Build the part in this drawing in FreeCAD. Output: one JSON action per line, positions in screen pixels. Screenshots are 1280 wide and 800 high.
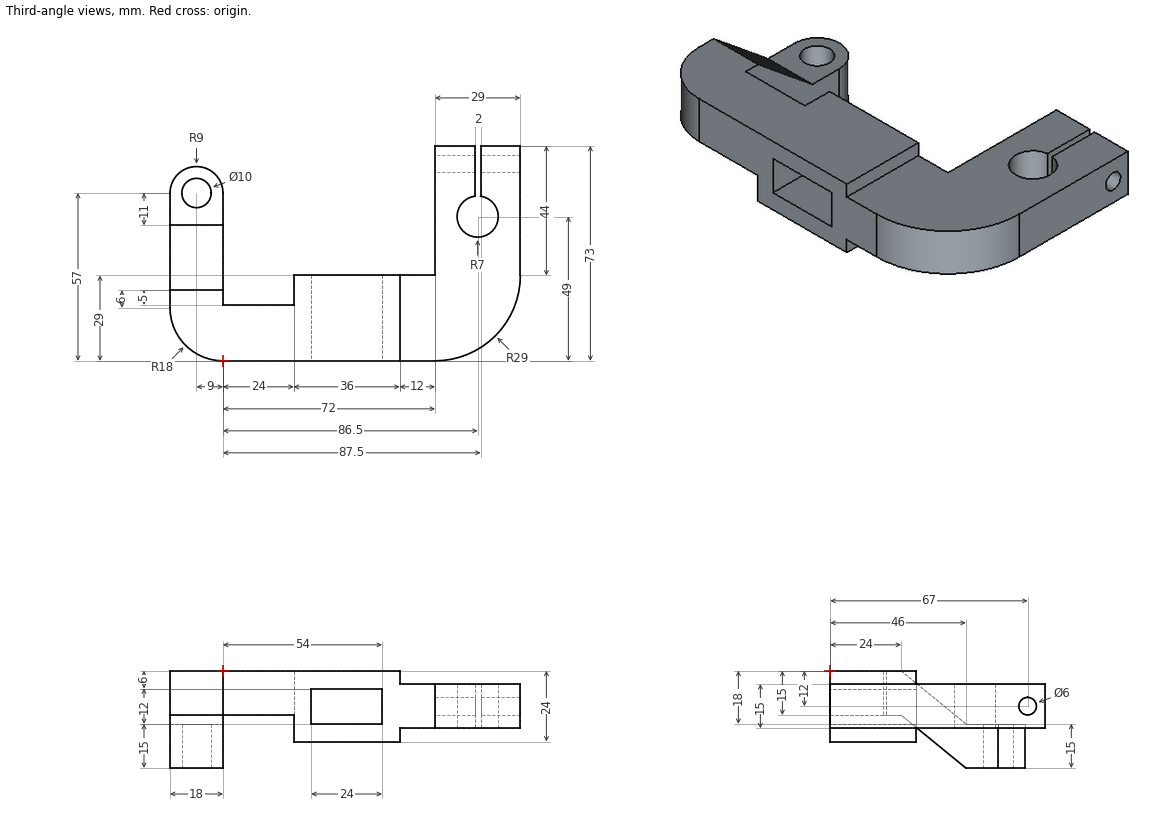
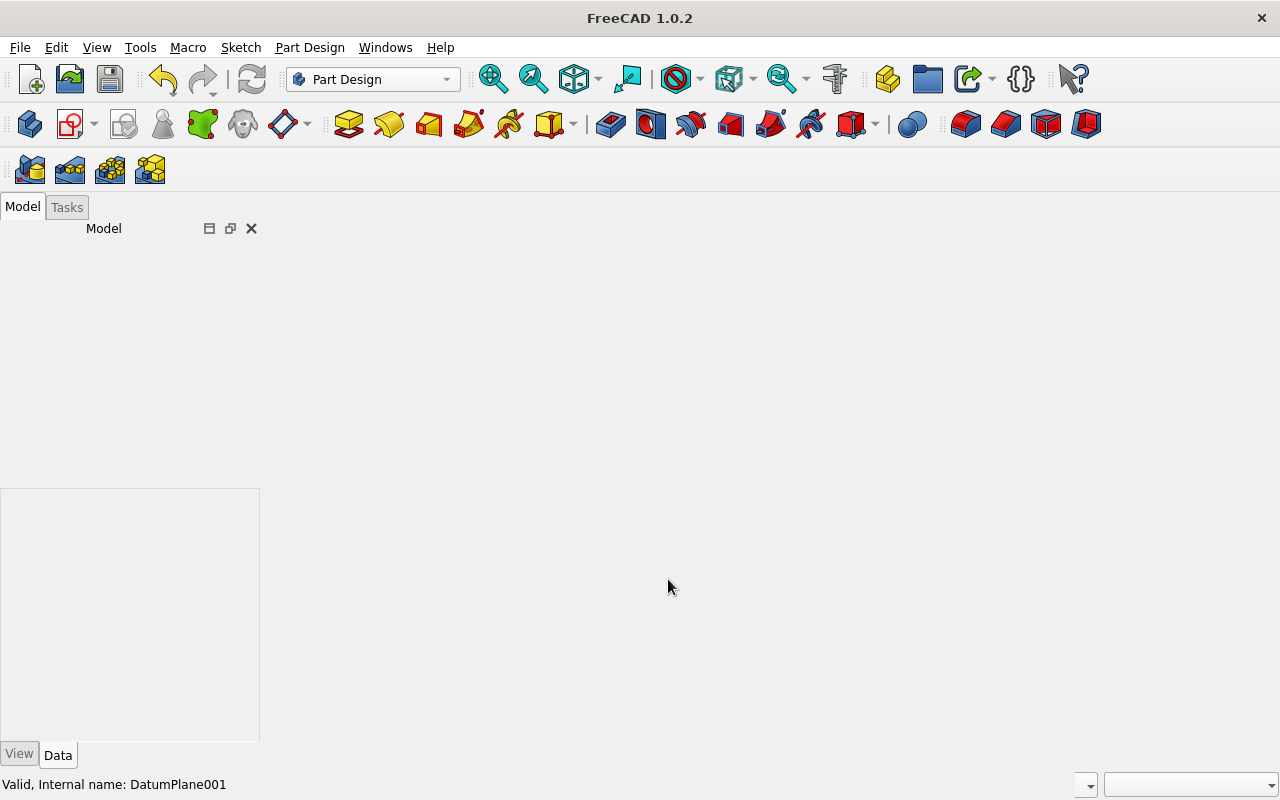
{"action": "key", "text": "ctrl+n"}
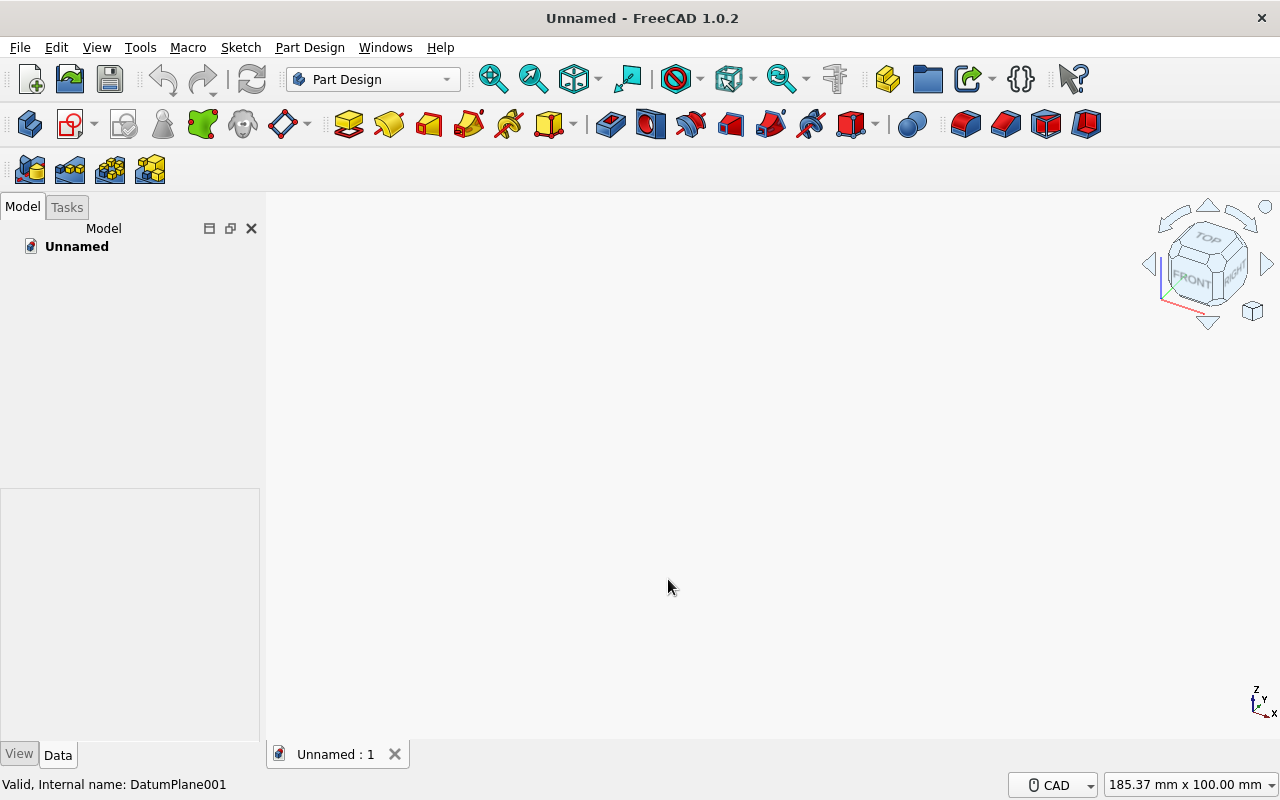
{"action": "left_click", "coordinate": [70, 124]}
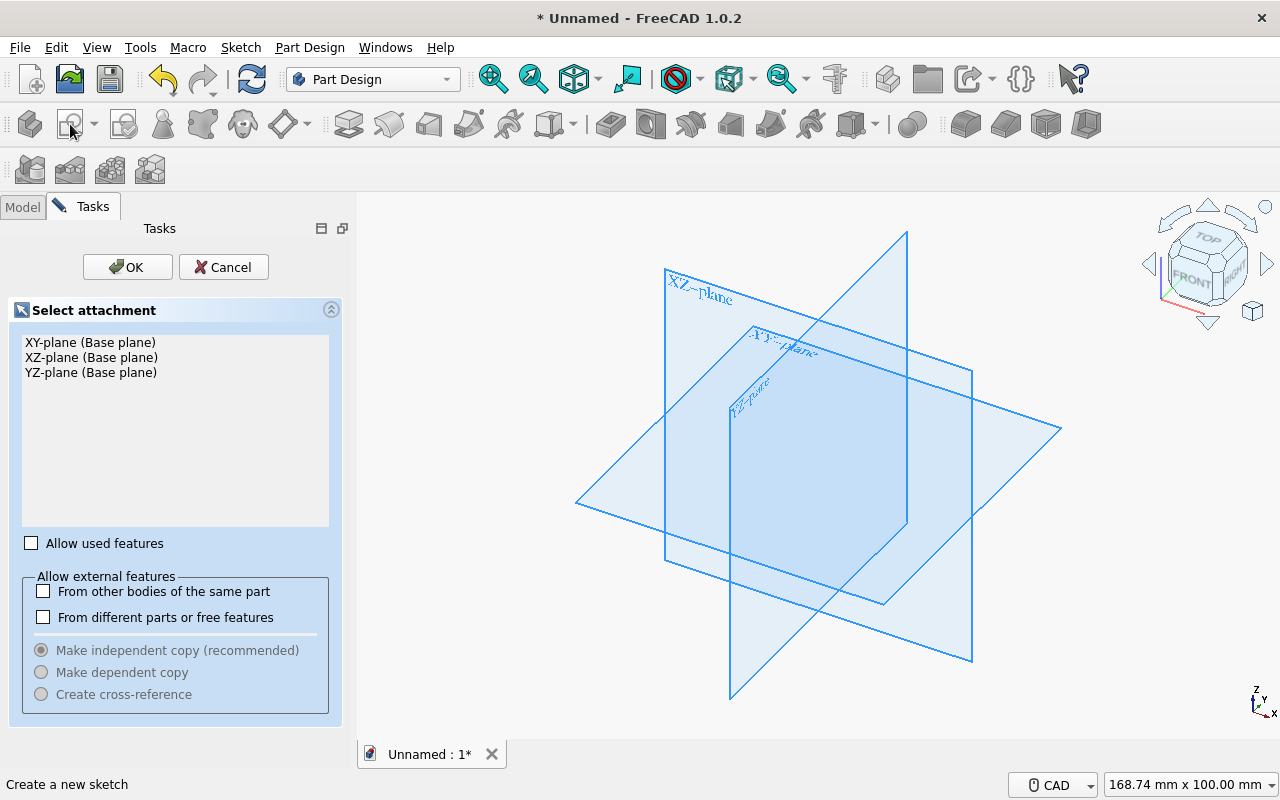
{"action": "left_click", "coordinate": [82, 342]}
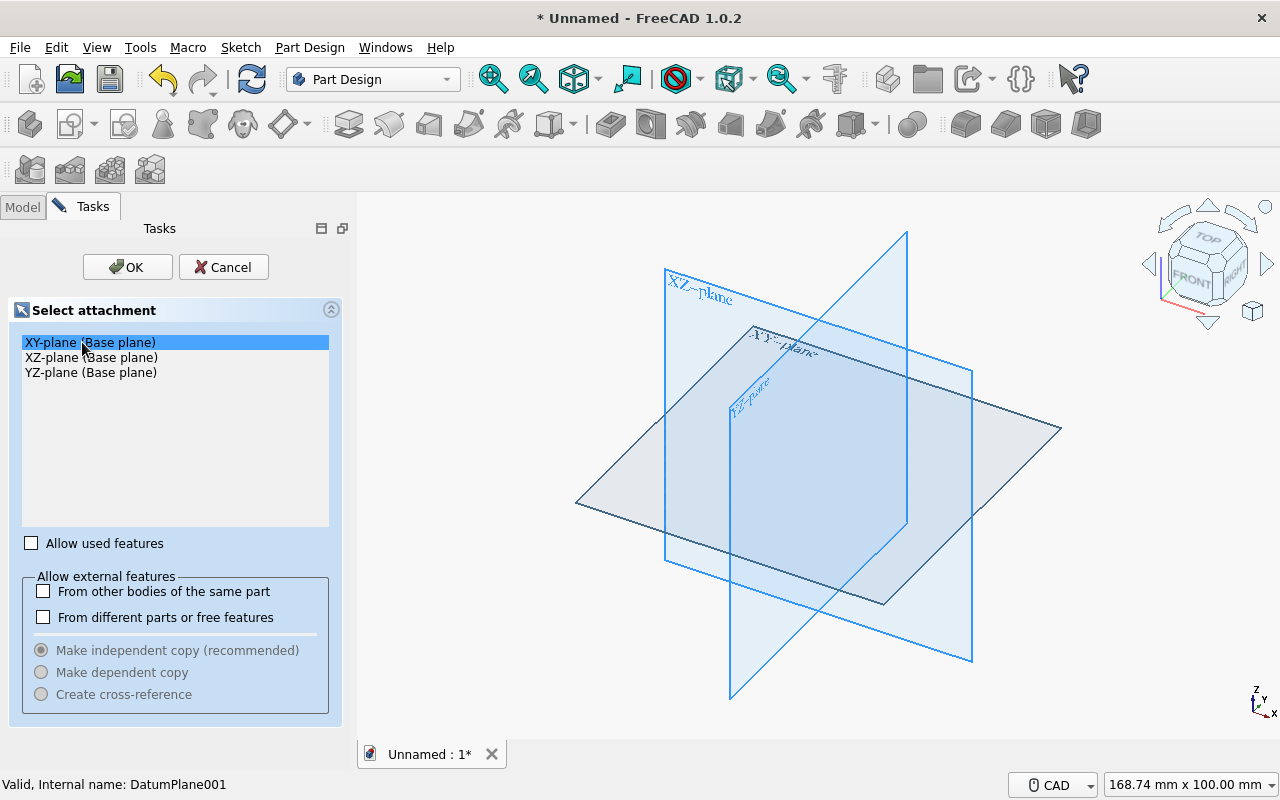
{"action": "left_click", "coordinate": [128, 267]}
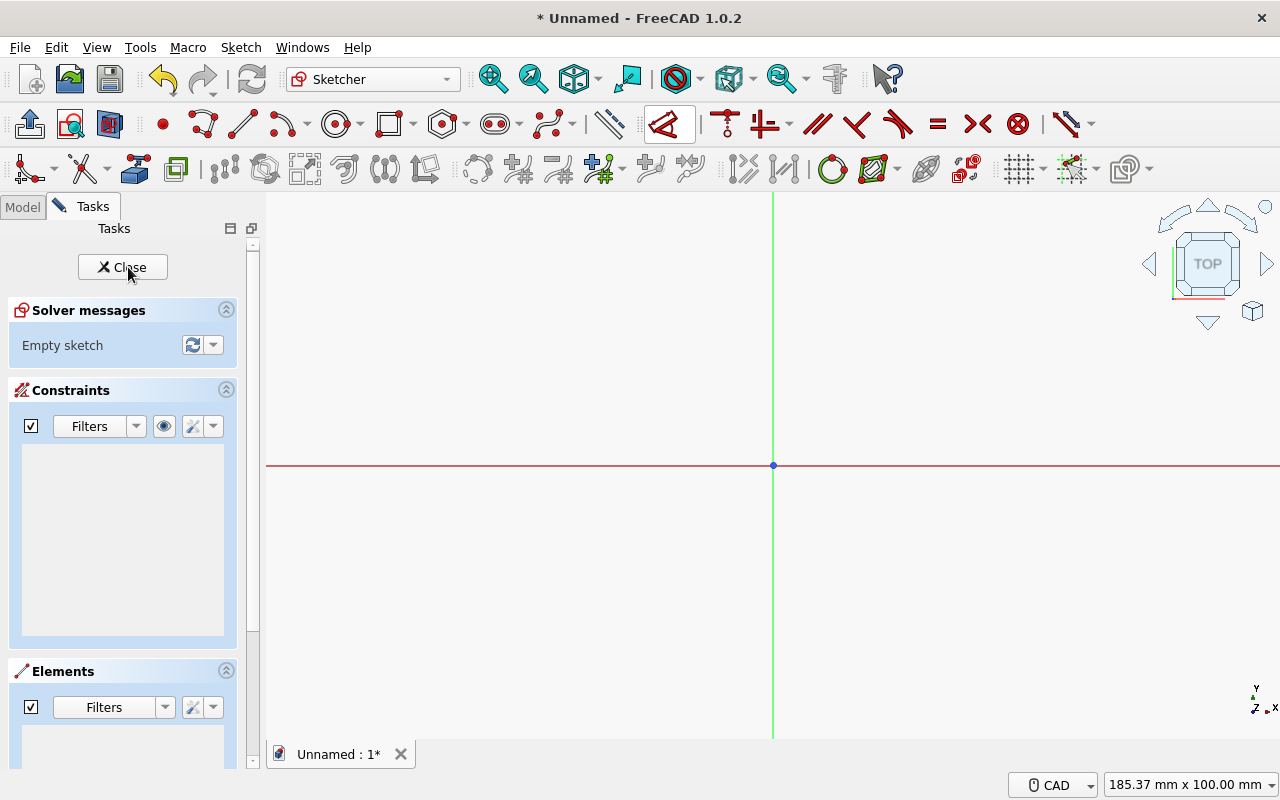
{"action": "scroll", "coordinate": [839, 362], "scroll_direction": "up", "scroll_amount": 5}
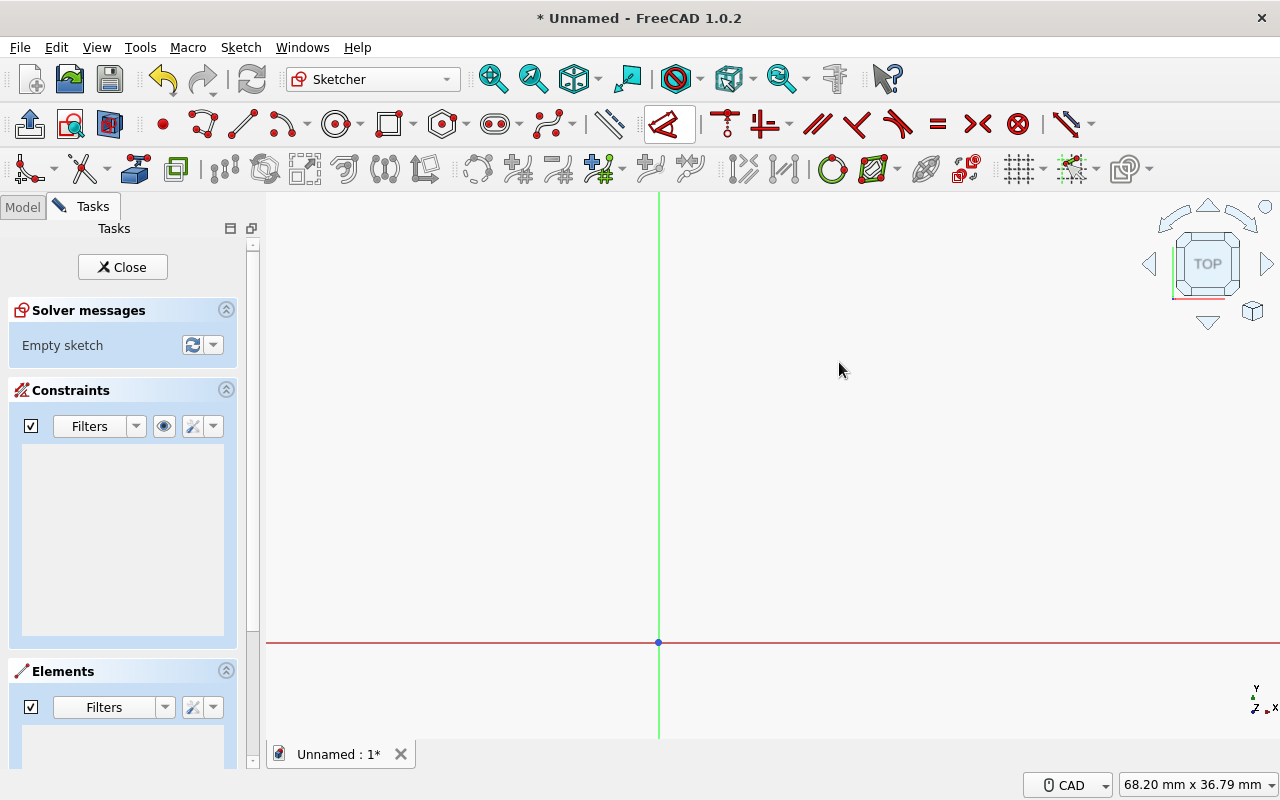
{"action": "left_click", "coordinate": [204, 124]}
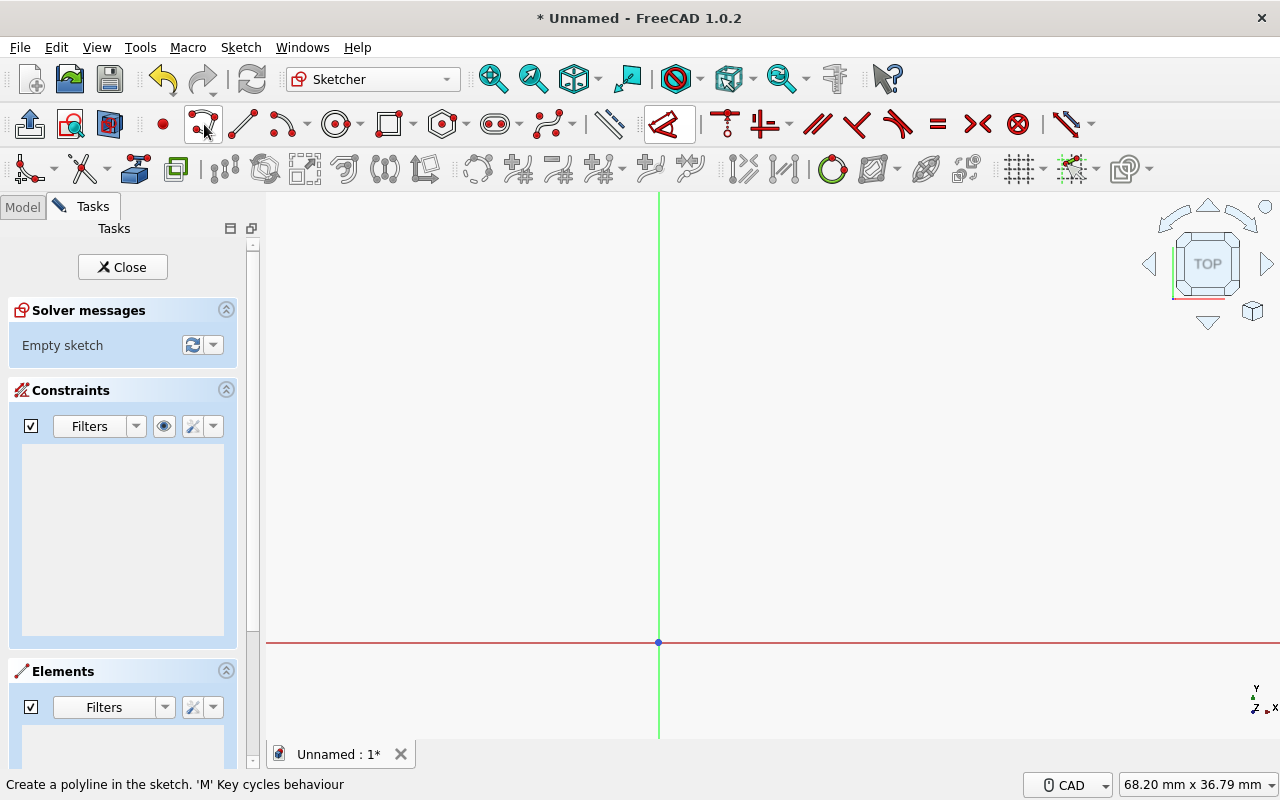
{"action": "left_click", "coordinate": [659, 643]}
{"action": "left_click", "coordinate": [1015, 634]}
{"action": "left_click", "coordinate": [1015, 360]}
{"action": "left_click", "coordinate": [659, 360]}
{"action": "left_click", "coordinate": [668, 286]}
{"action": "left_click", "coordinate": [391, 286]}
{"action": "left_click", "coordinate": [391, 375]}
{"action": "right_click", "coordinate": [391, 375]}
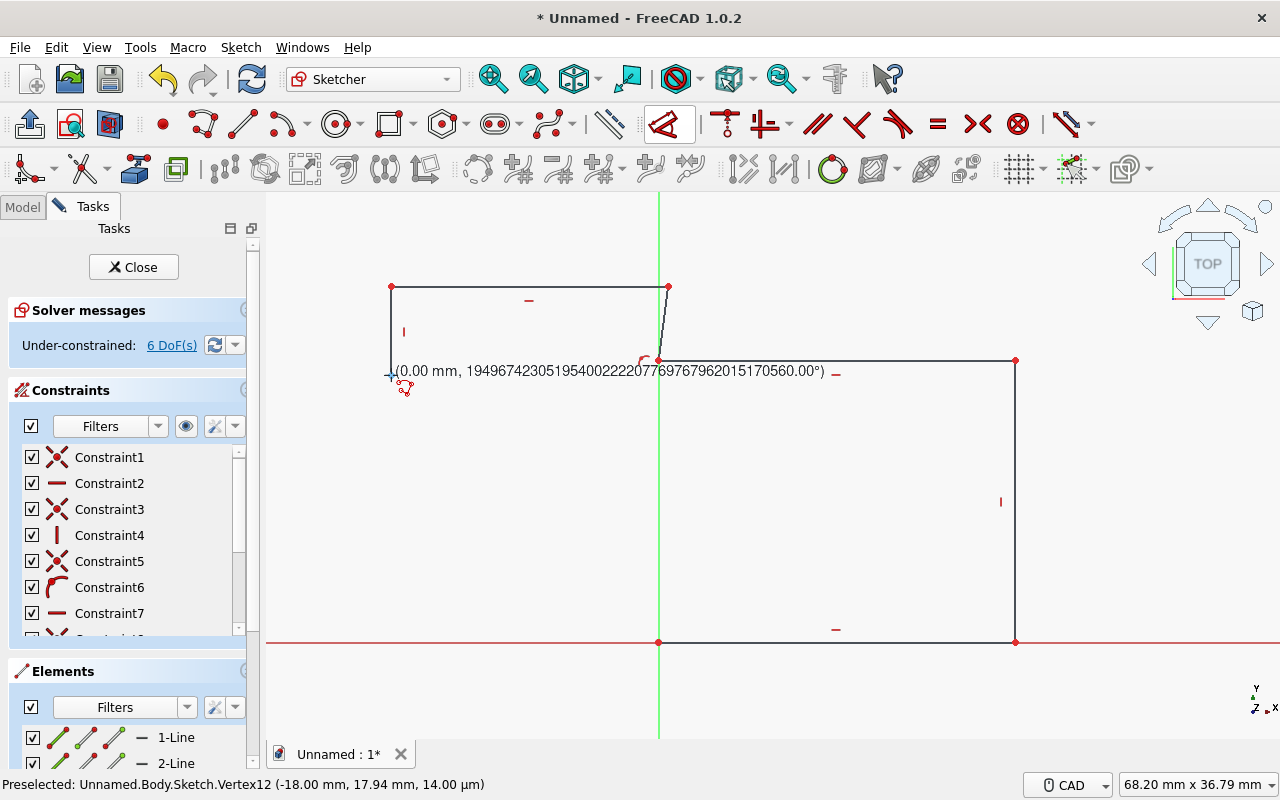
{"action": "key", "text": "g 3 a"}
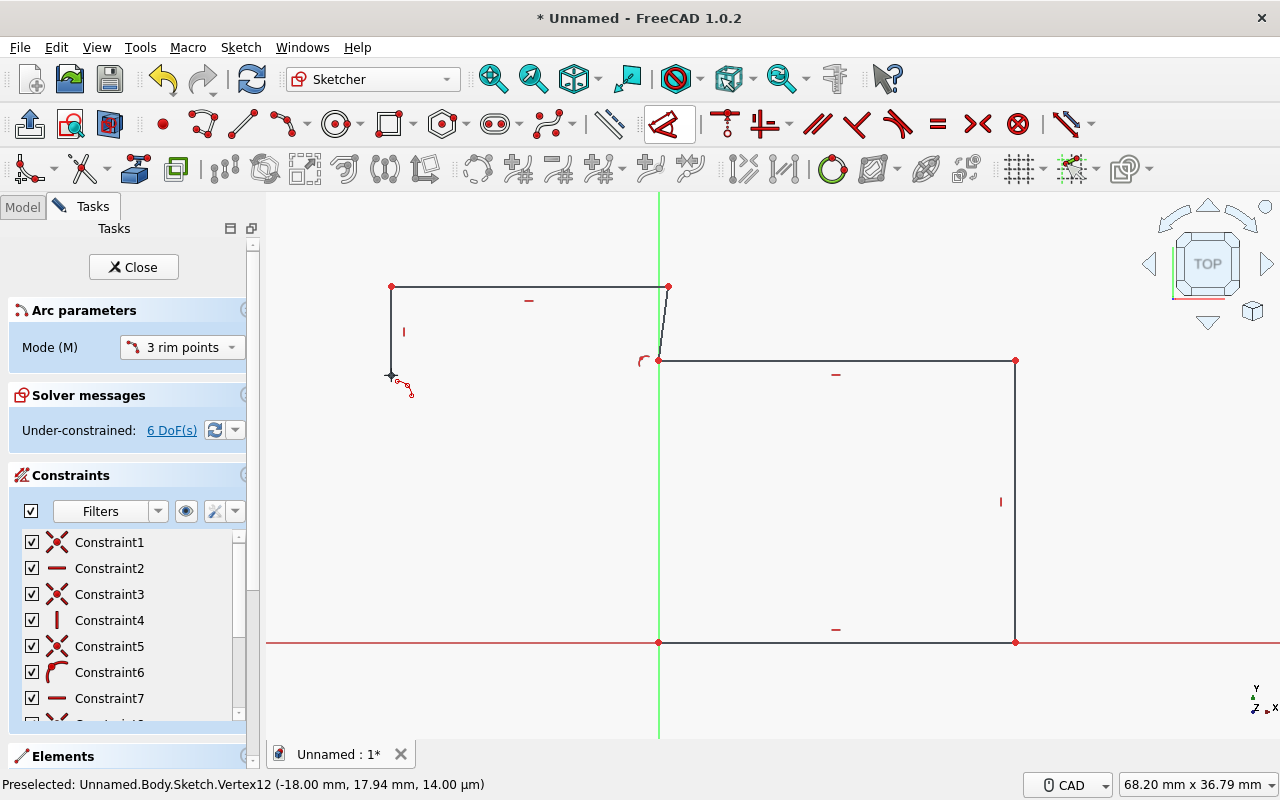
{"action": "left_click", "coordinate": [391, 376]}
{"action": "left_click", "coordinate": [659, 643]}
{"action": "left_click", "coordinate": [469, 564]}
{"action": "key", "text": "Escape"}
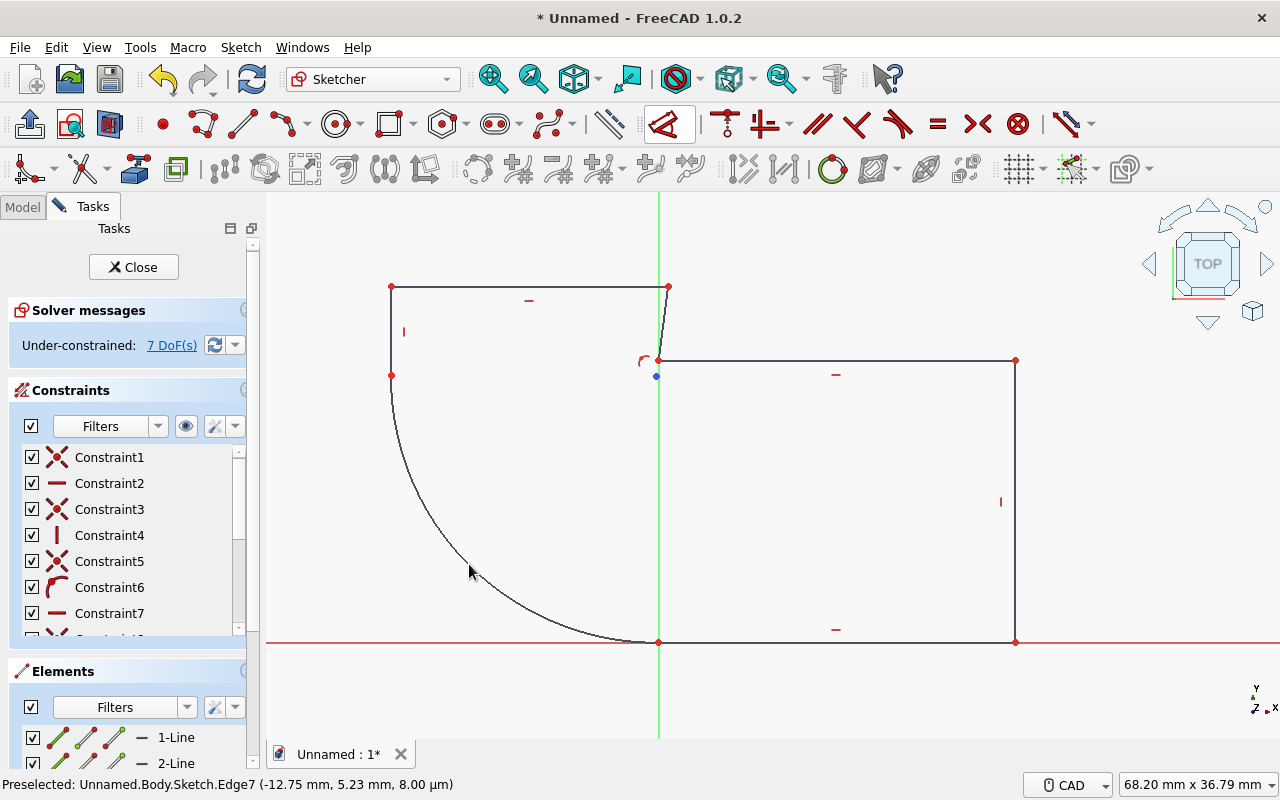
{"action": "left_click", "coordinate": [766, 643]}